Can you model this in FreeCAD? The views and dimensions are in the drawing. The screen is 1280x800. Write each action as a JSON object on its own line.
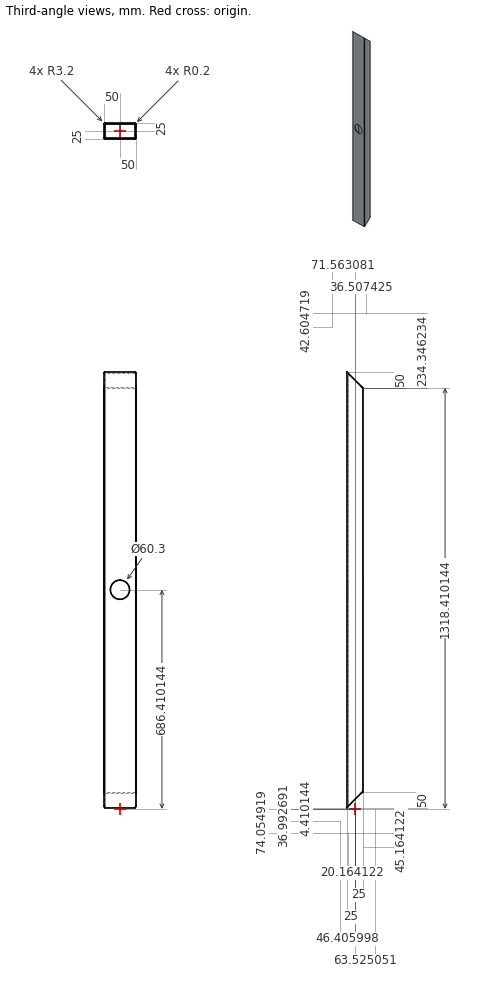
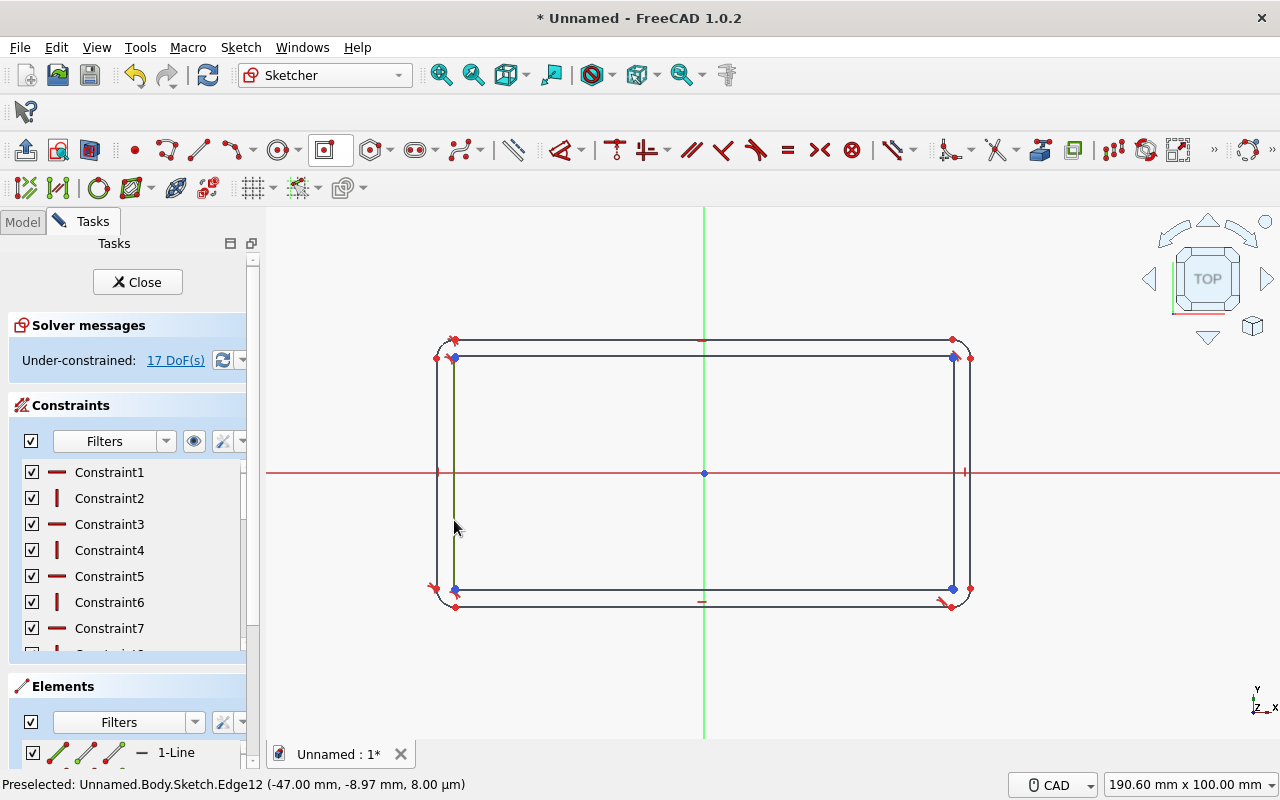
{"action": "scroll", "coordinate": [454, 357], "scroll_direction": "up", "scroll_amount": 14}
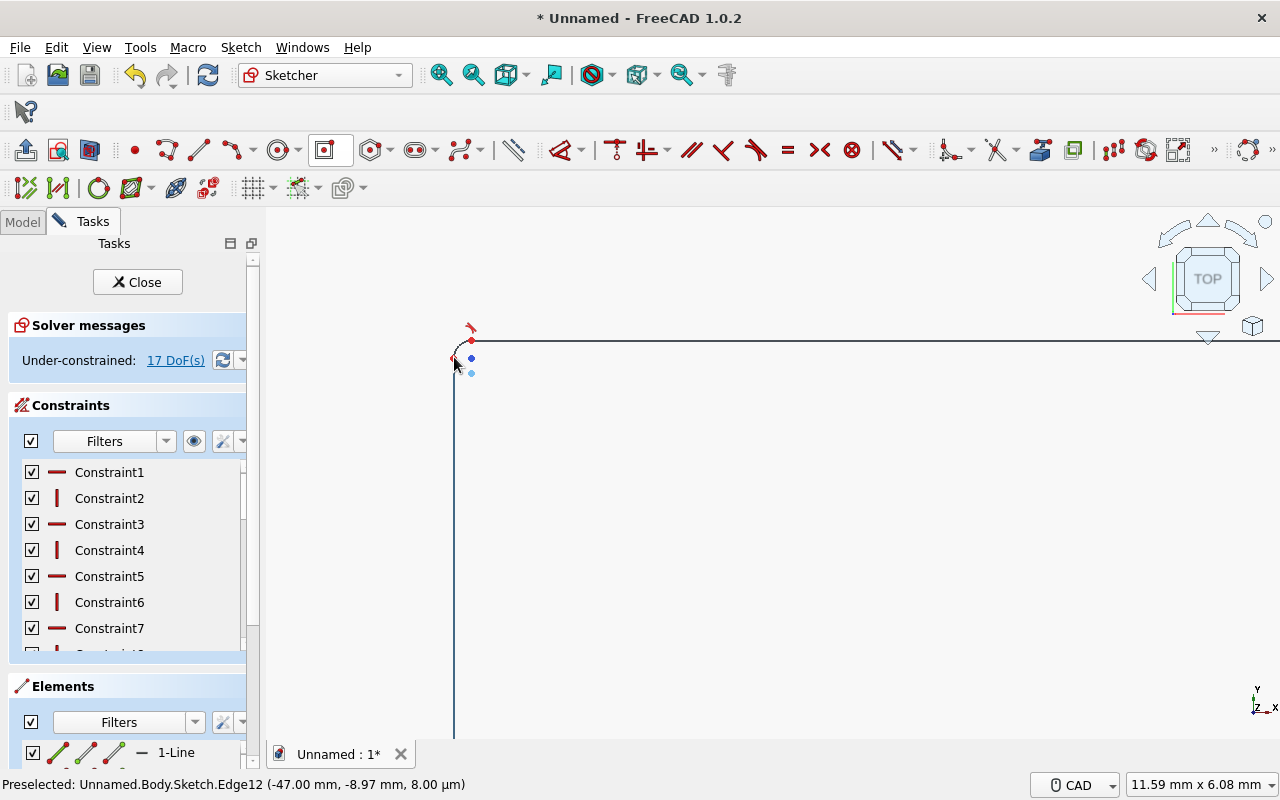
{"action": "left_click", "coordinate": [459, 346]}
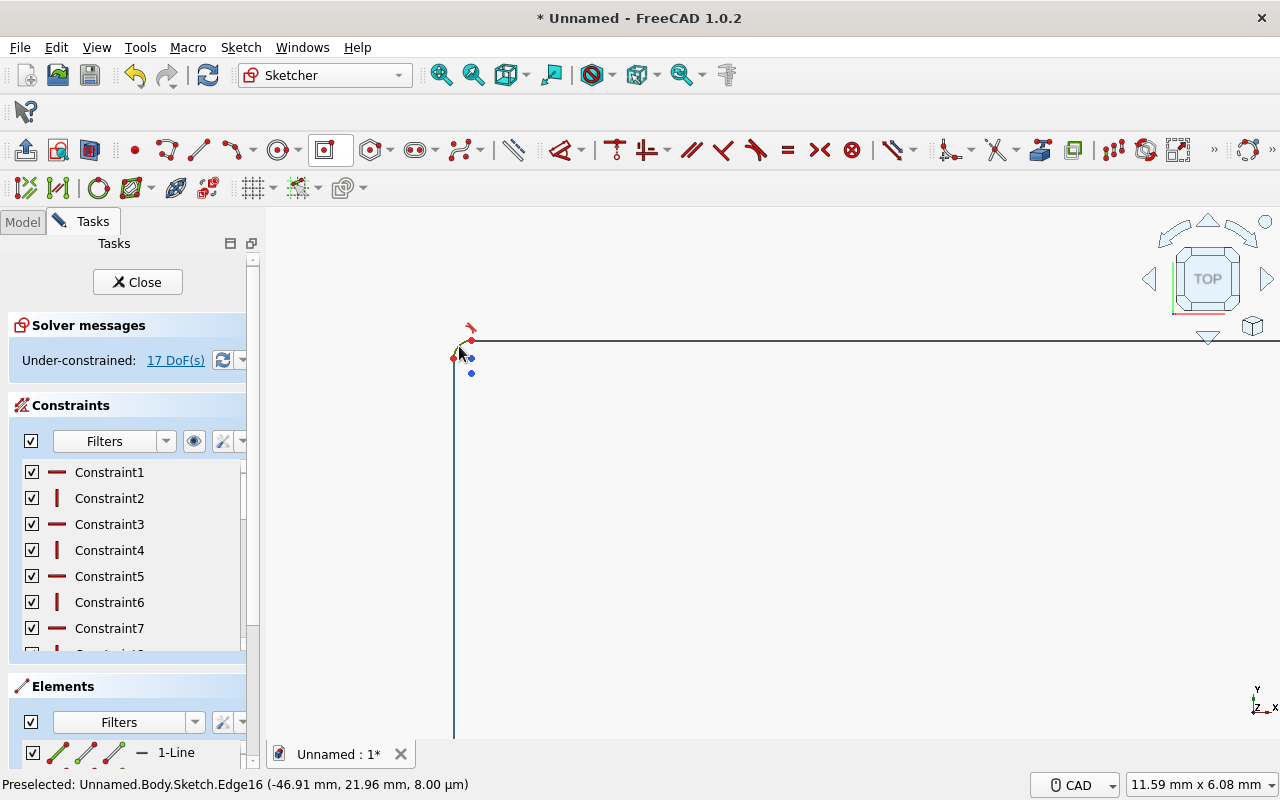
{"action": "key", "text": "t"}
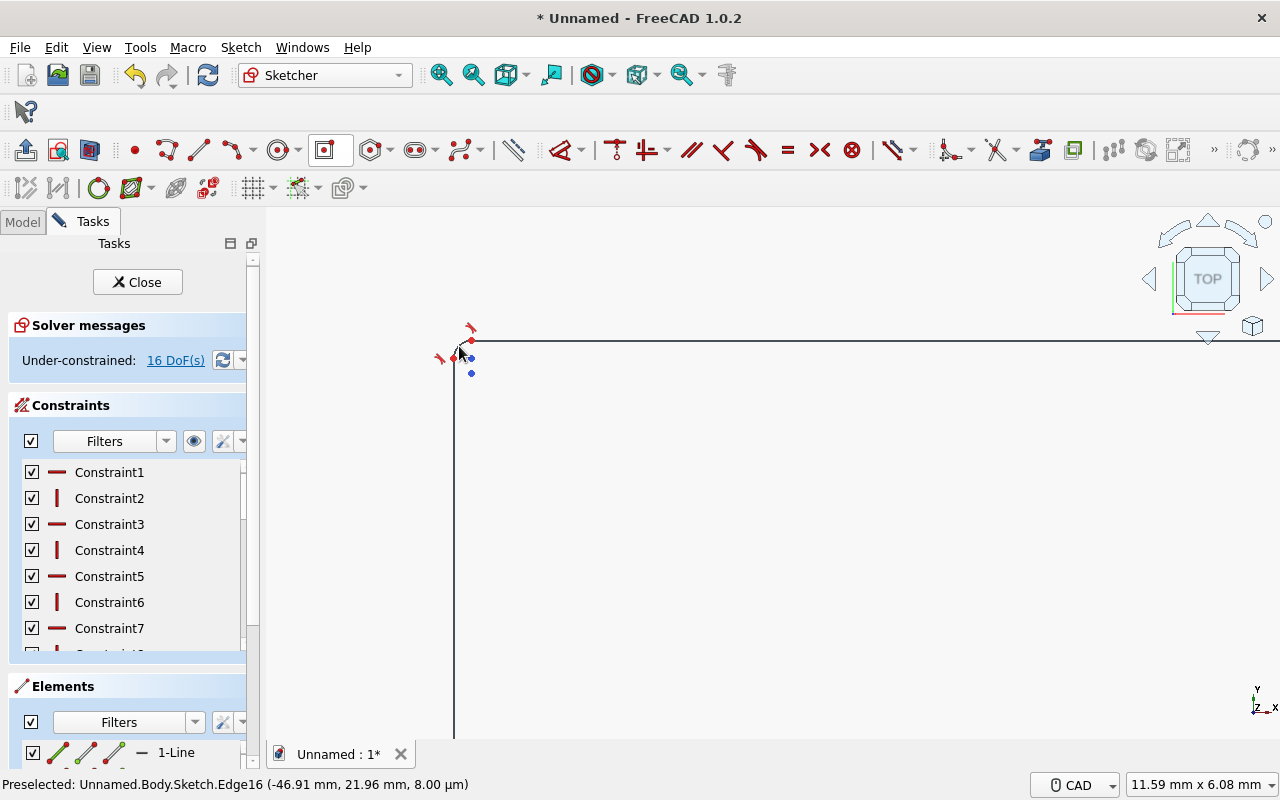
{"action": "scroll", "coordinate": [454, 357], "scroll_direction": "down", "scroll_amount": 14}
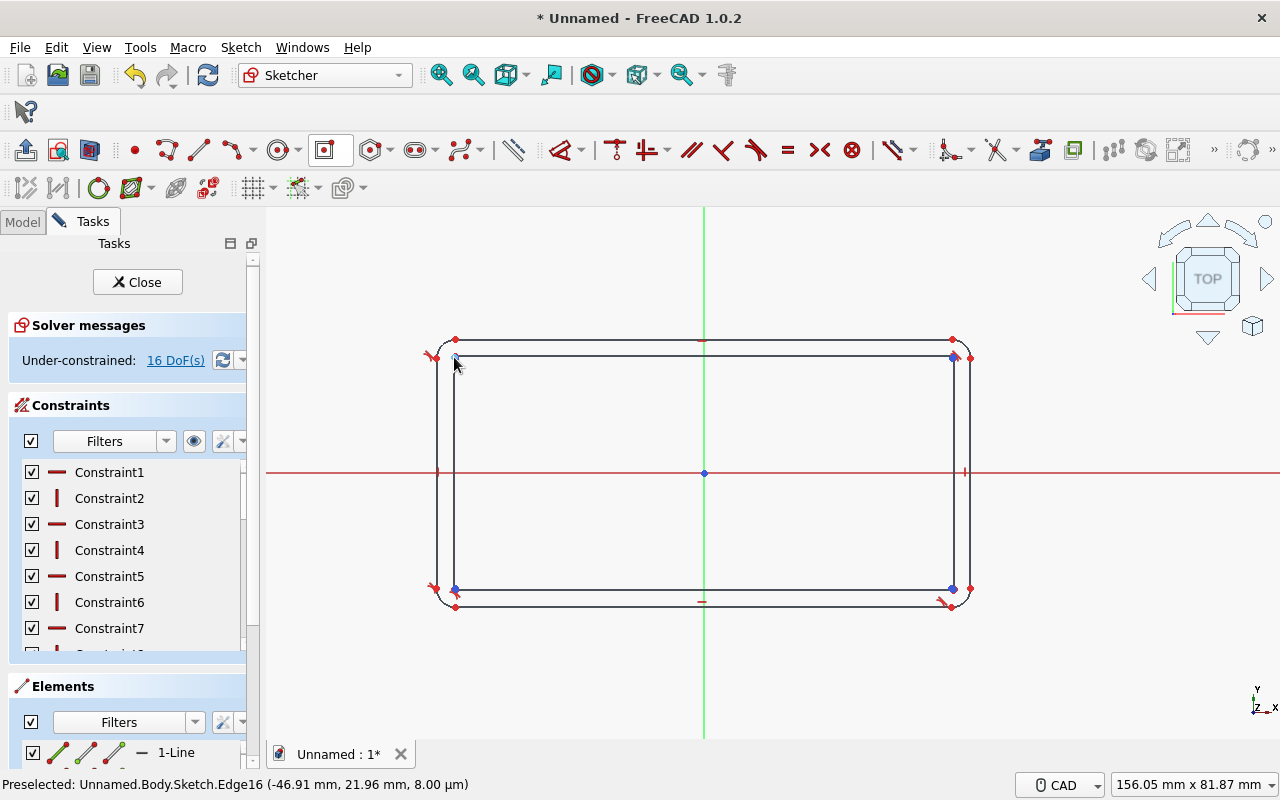
{"action": "scroll", "coordinate": [969, 350], "scroll_direction": "up", "scroll_amount": 3}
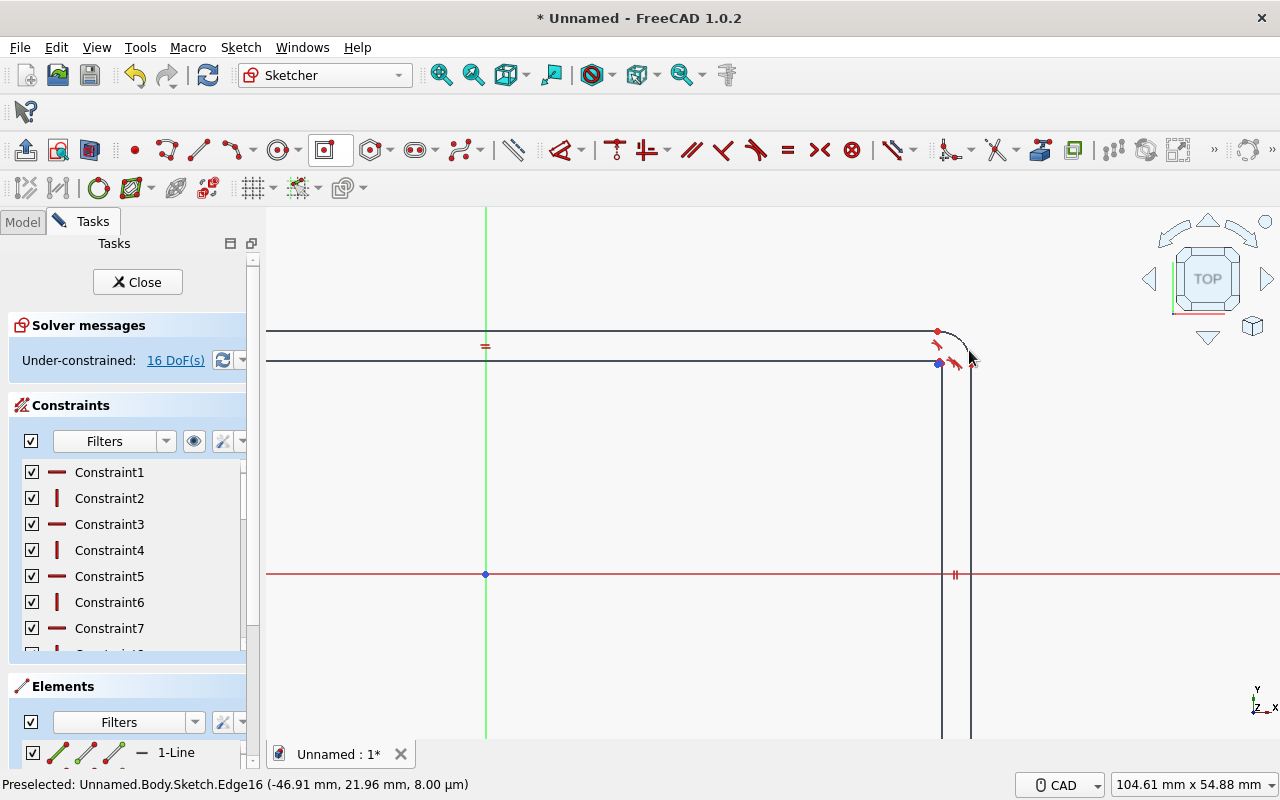
{"action": "left_click", "coordinate": [968, 350]}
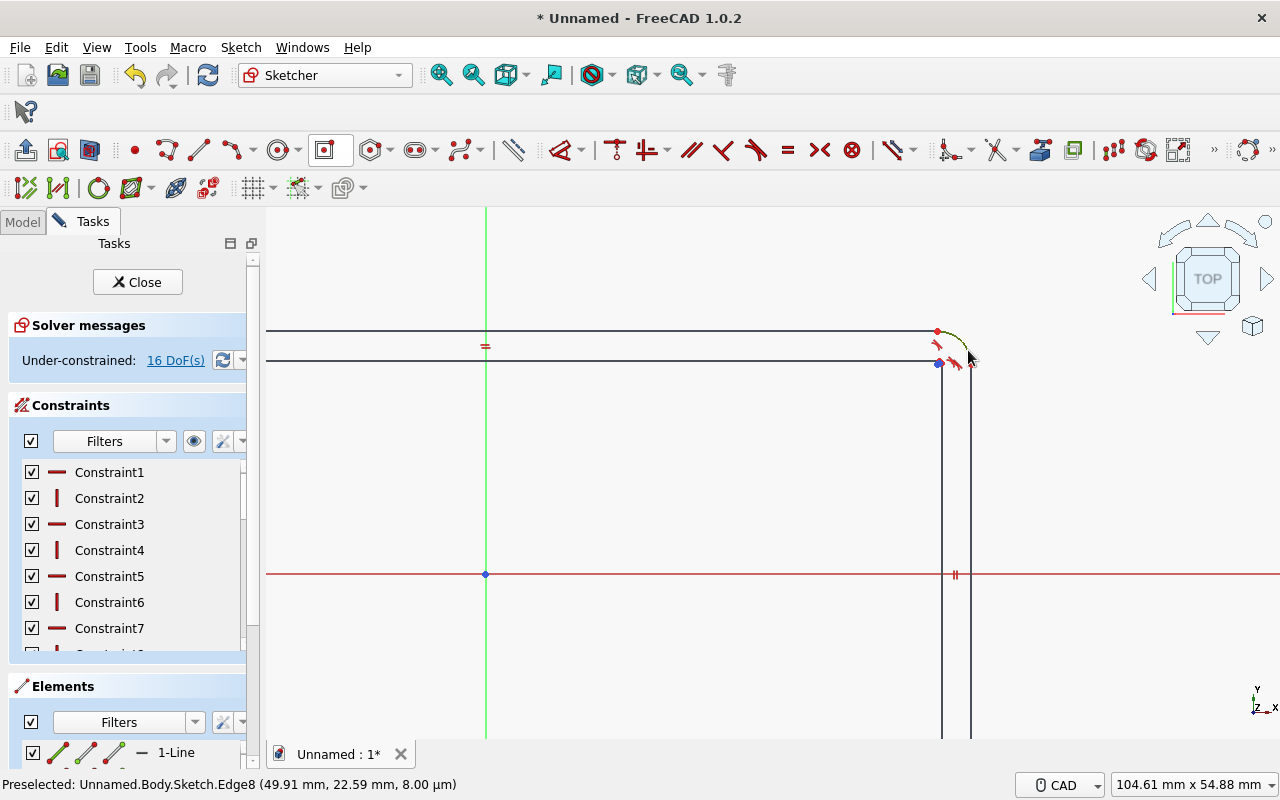
{"action": "scroll", "coordinate": [941, 362], "scroll_direction": "up", "scroll_amount": 11}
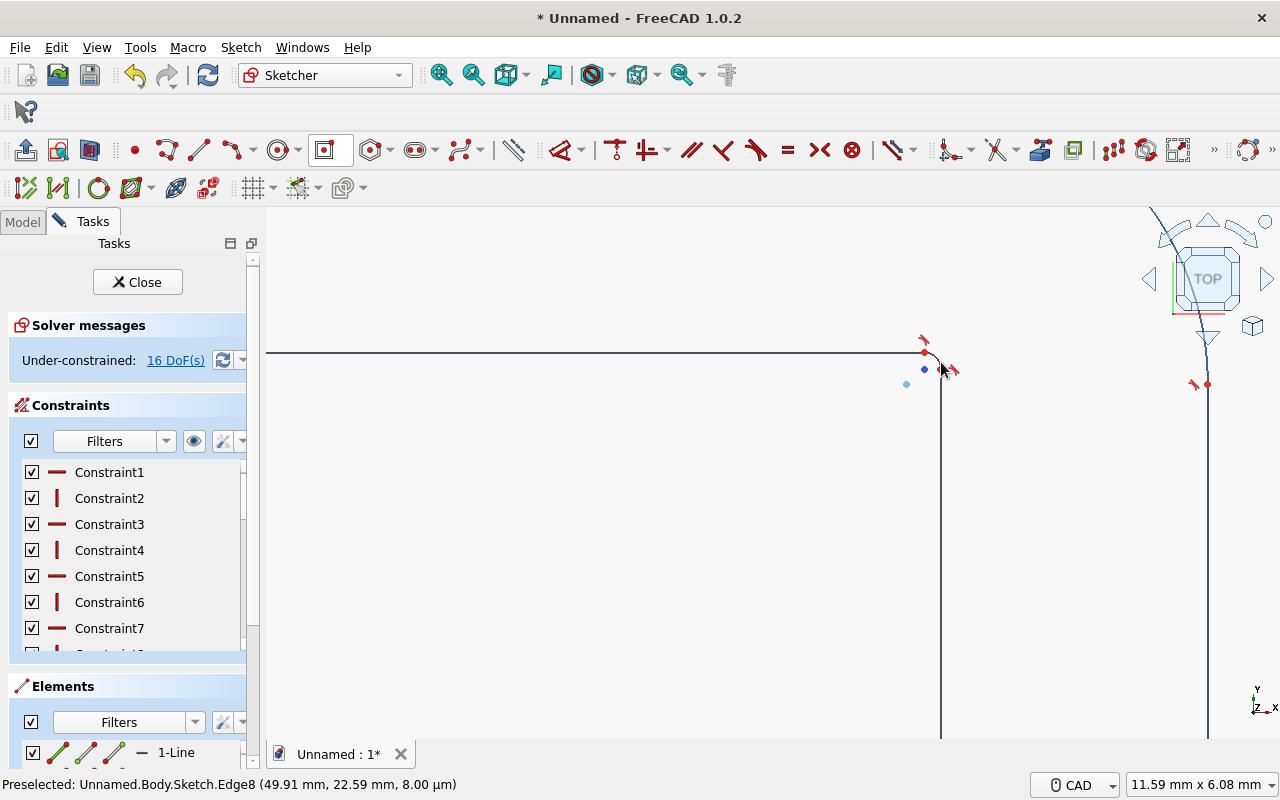
{"action": "left_click", "coordinate": [936, 357]}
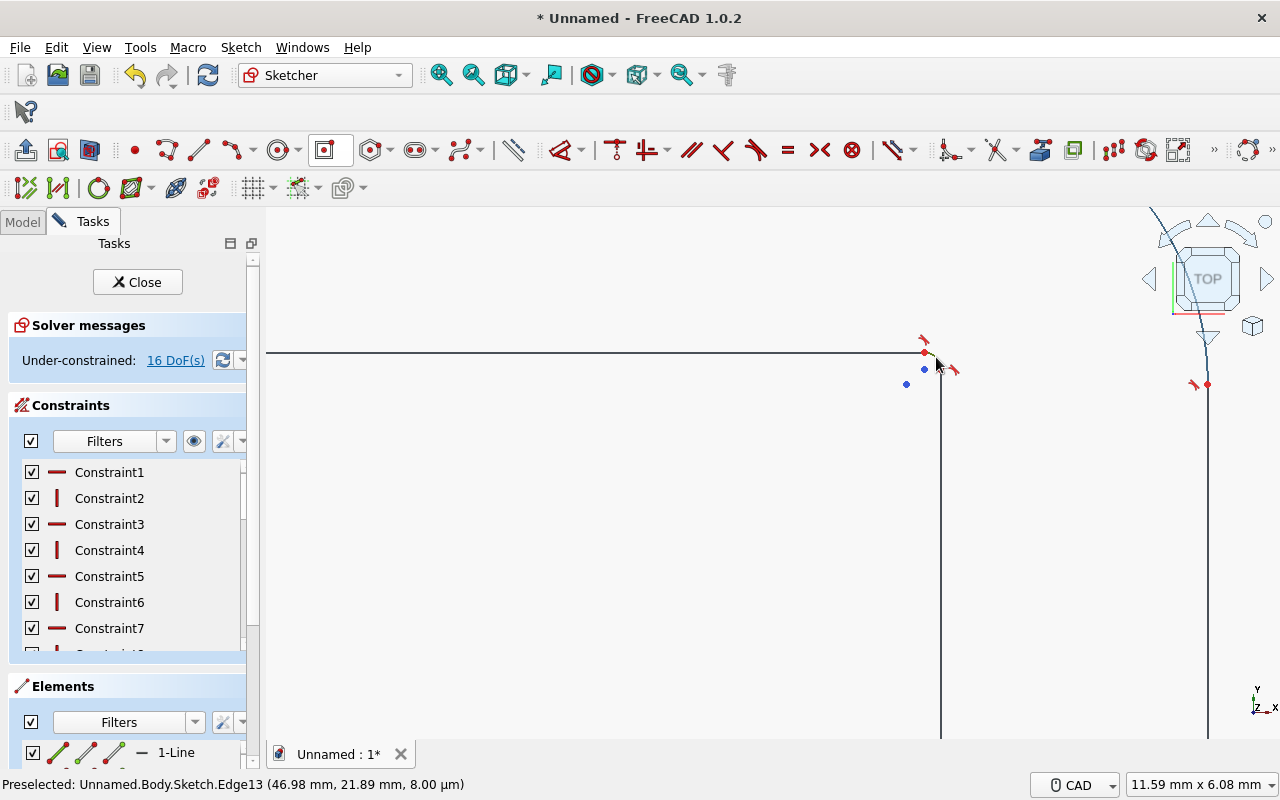
{"action": "left_click", "coordinate": [616, 150]}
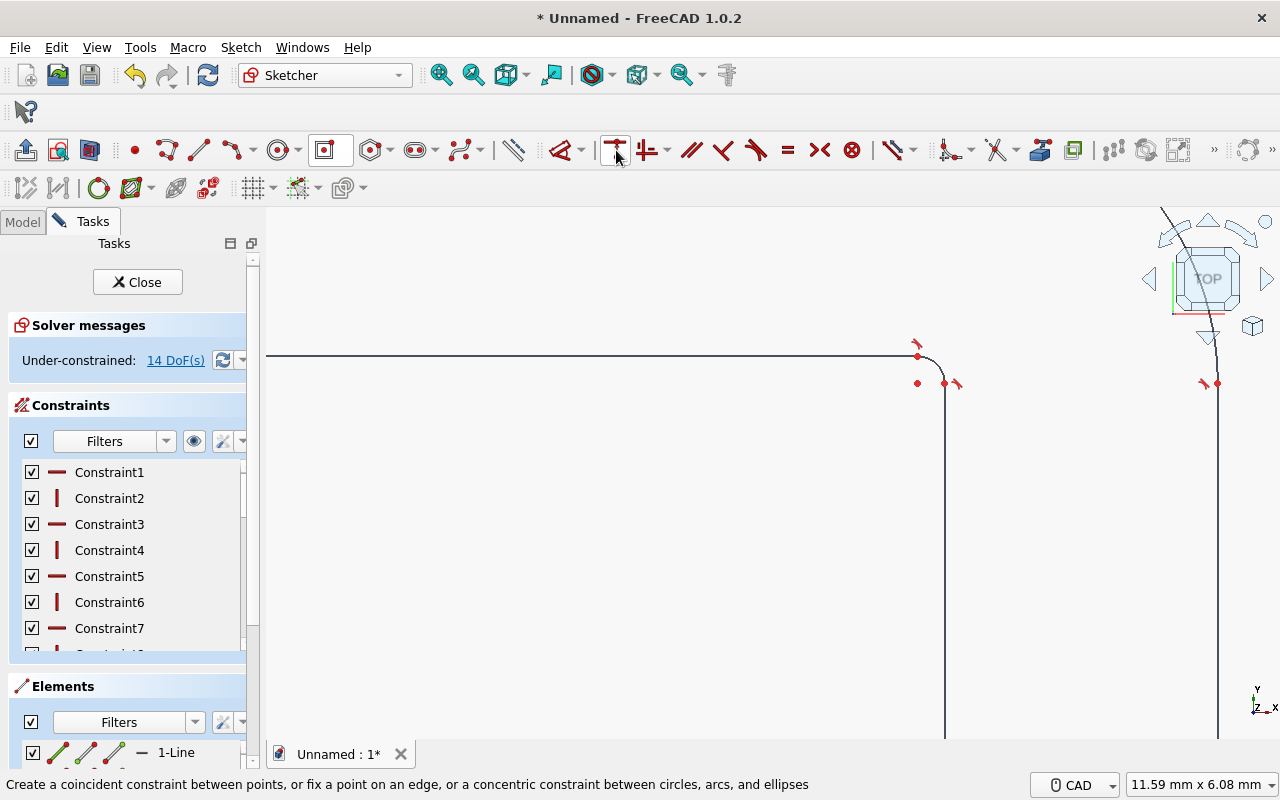
{"action": "scroll", "coordinate": [955, 356], "scroll_direction": "down", "scroll_amount": 14}